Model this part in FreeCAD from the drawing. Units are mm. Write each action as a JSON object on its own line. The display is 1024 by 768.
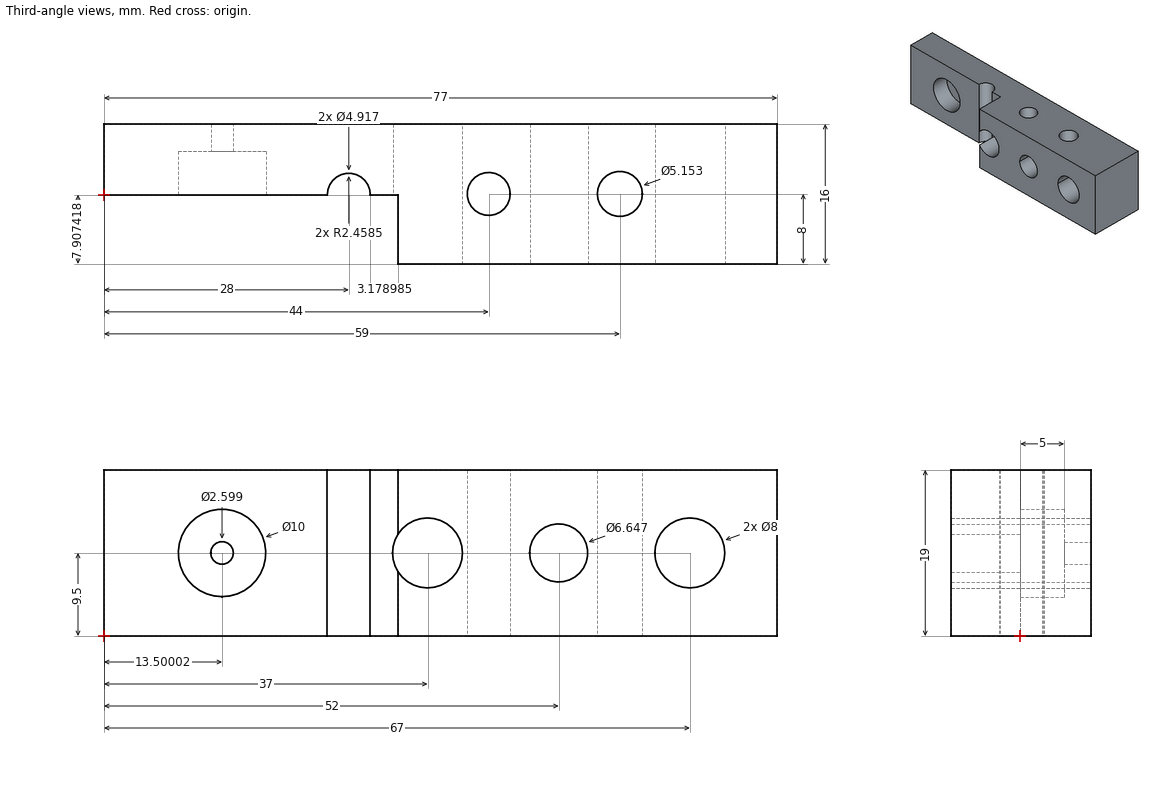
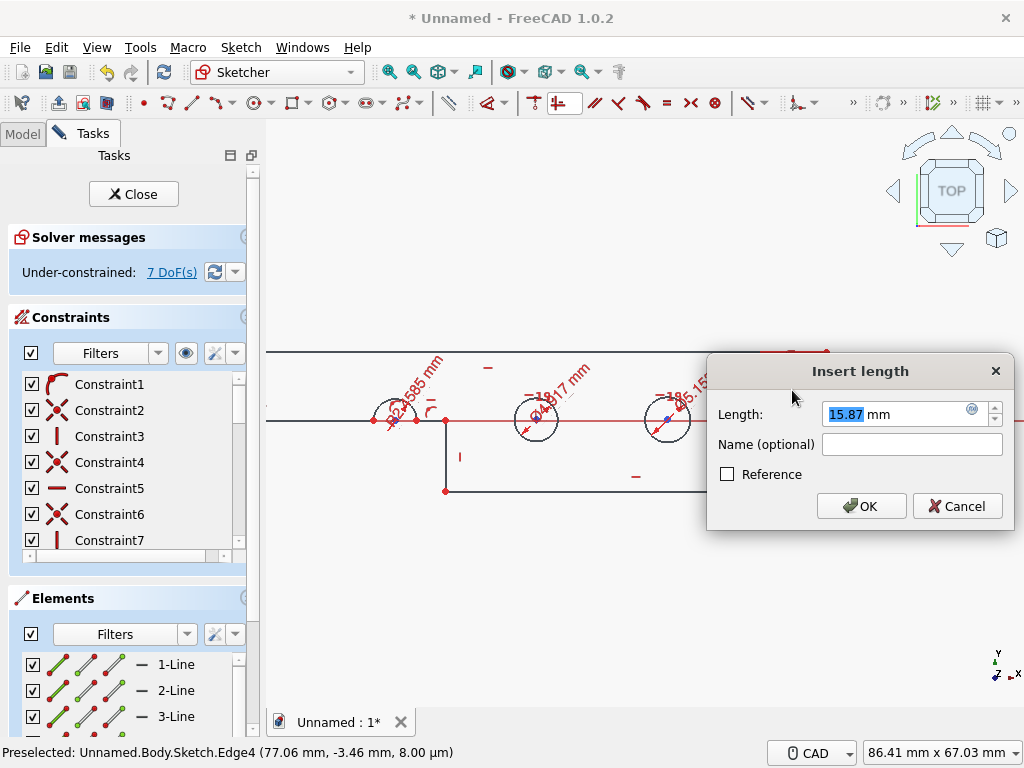
{"action": "type", "text": "16"}
{"action": "key", "text": "Return"}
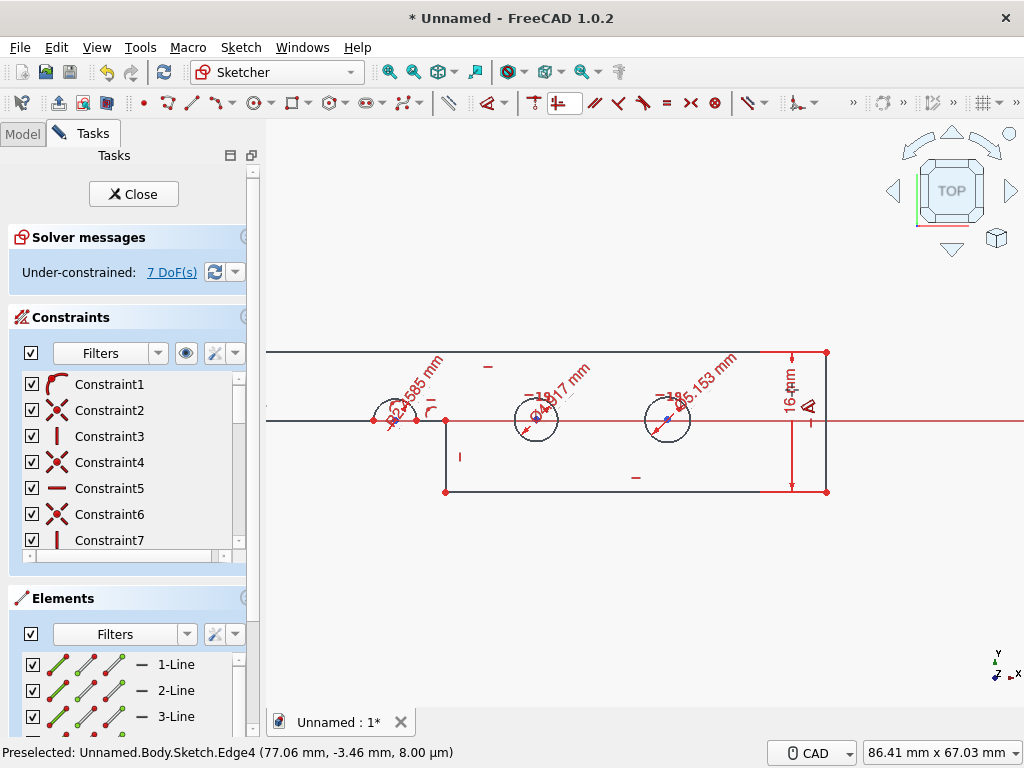
{"action": "left_click", "coordinate": [623, 352]}
{"action": "left_click", "coordinate": [560, 318]}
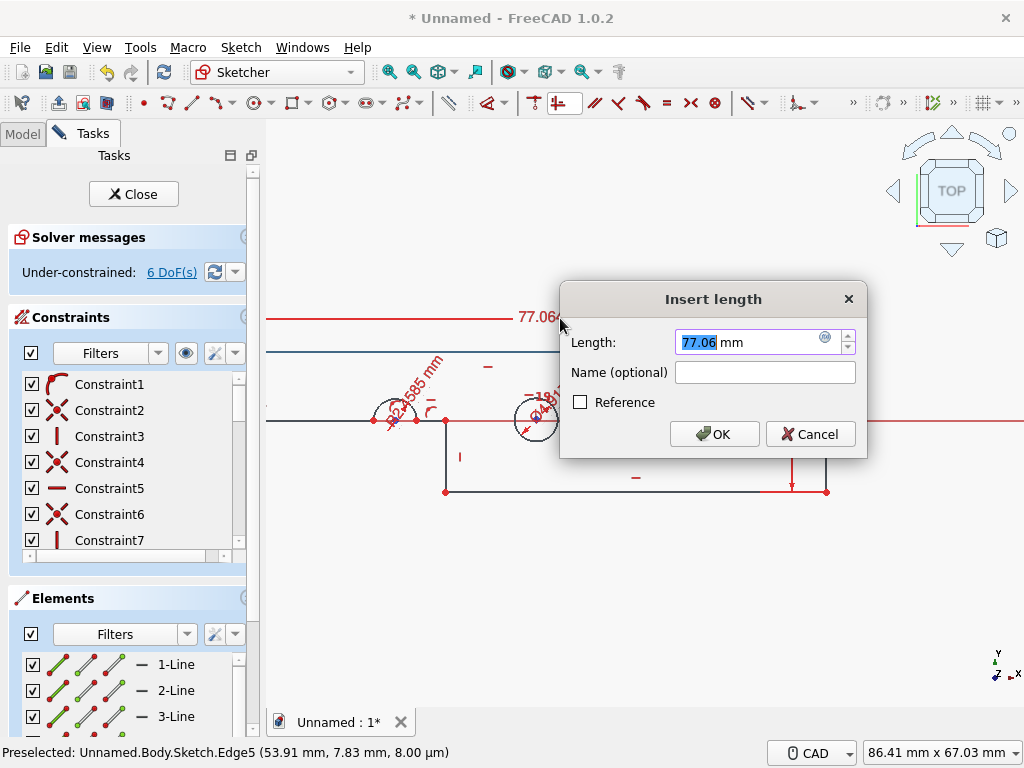
{"action": "type", "text": "77"}
{"action": "key", "text": "Return"}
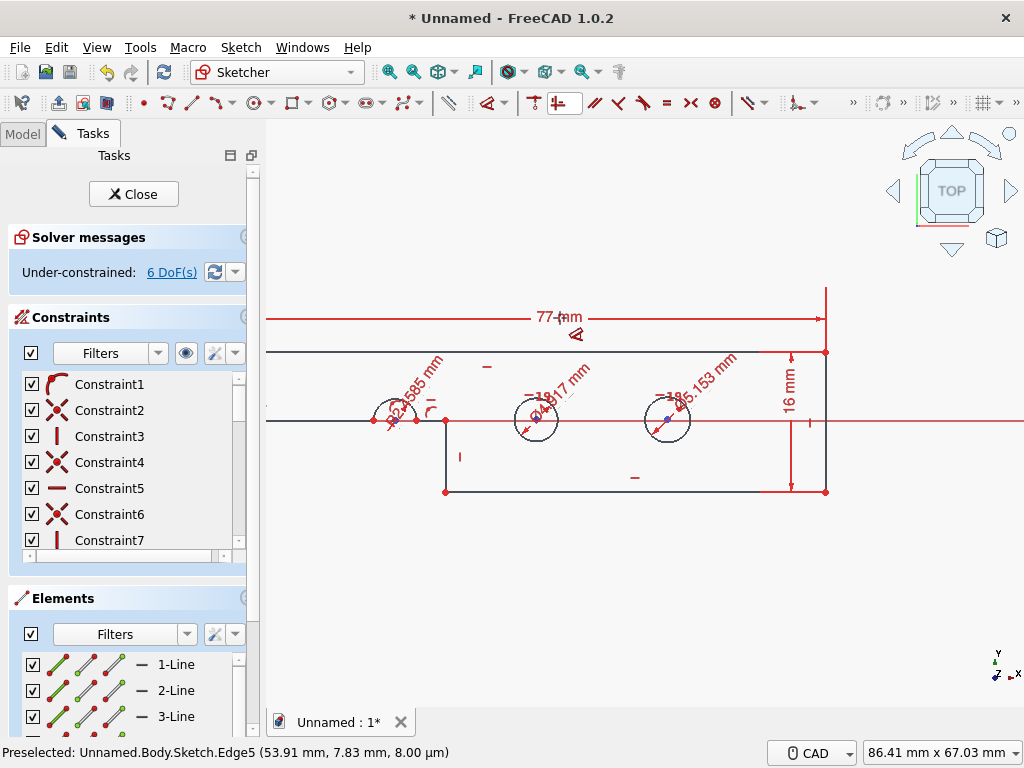
{"action": "left_click", "coordinate": [536, 420]}
{"action": "left_click", "coordinate": [415, 455]}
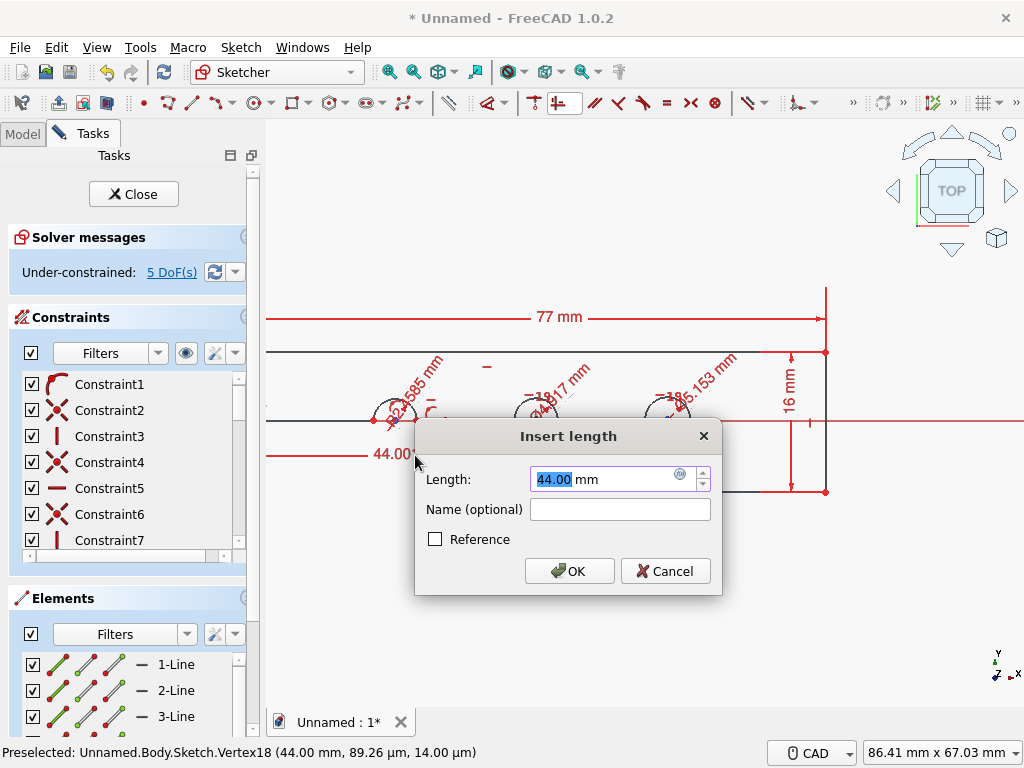
{"action": "type", "text": "44"}
{"action": "key", "text": "Return"}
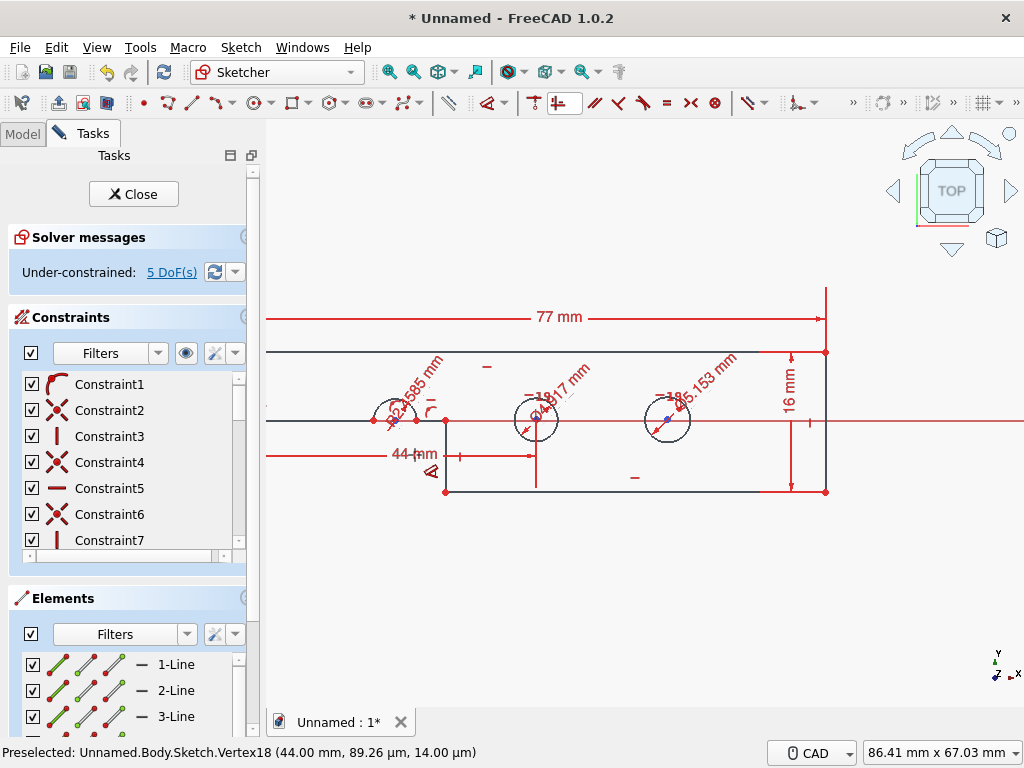
{"action": "left_click", "coordinate": [668, 420]}
{"action": "left_click", "coordinate": [567, 455]}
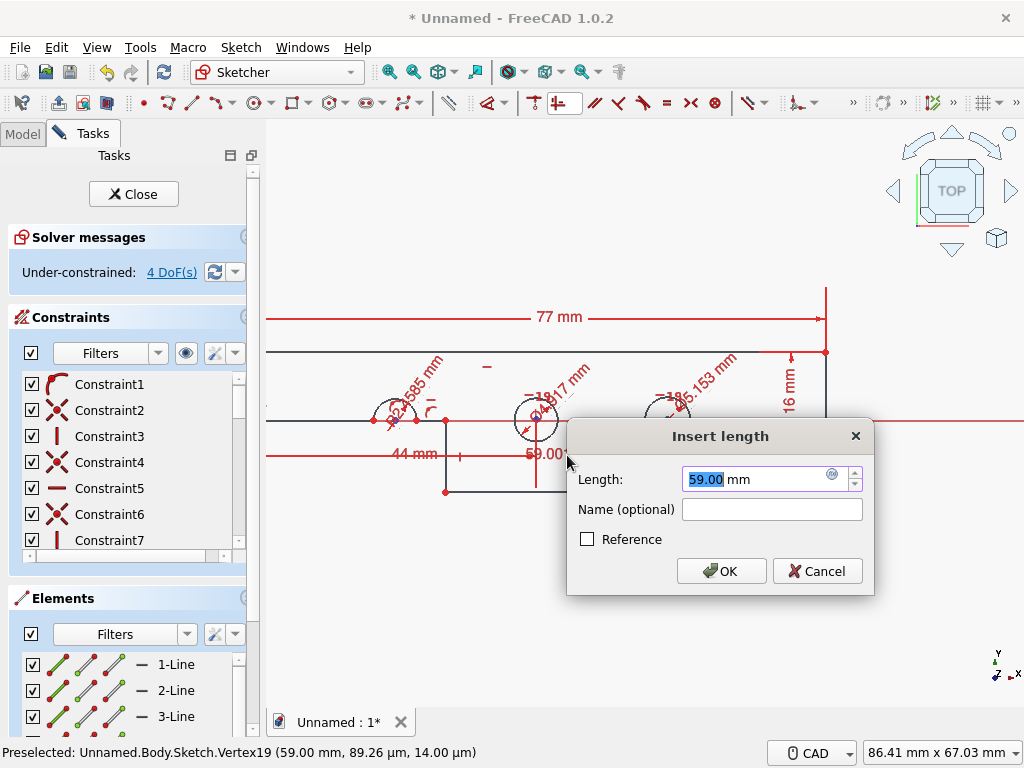
{"action": "type", "text": "59"}
{"action": "key", "text": "Return"}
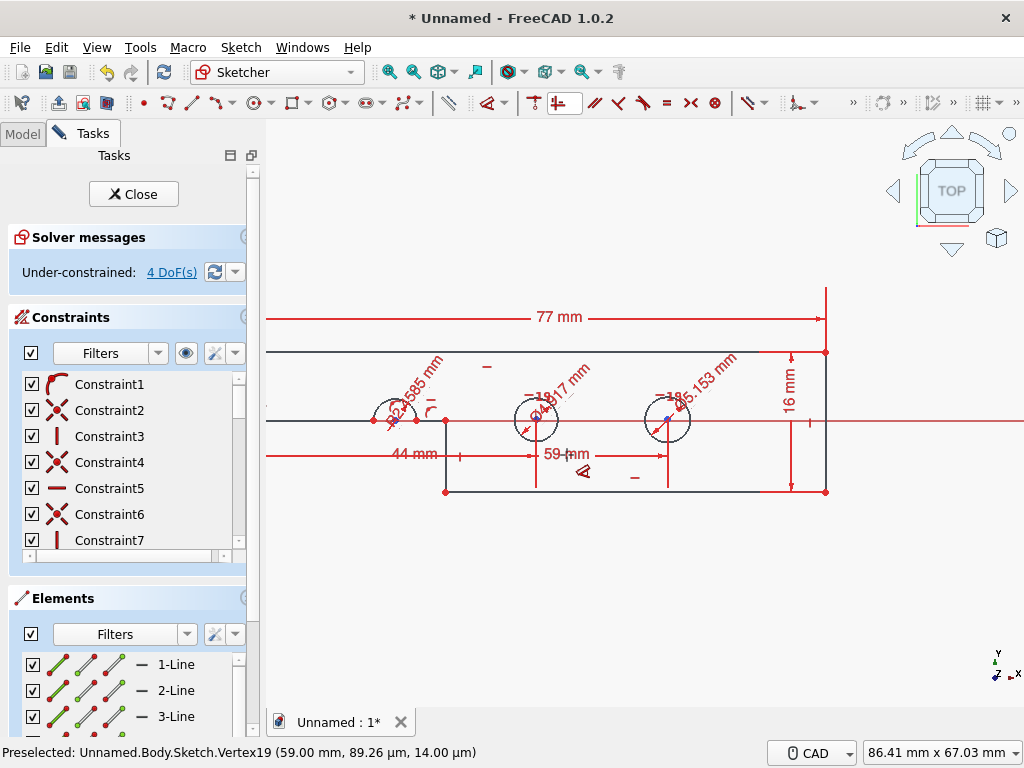
{"action": "left_click", "coordinate": [446, 492]}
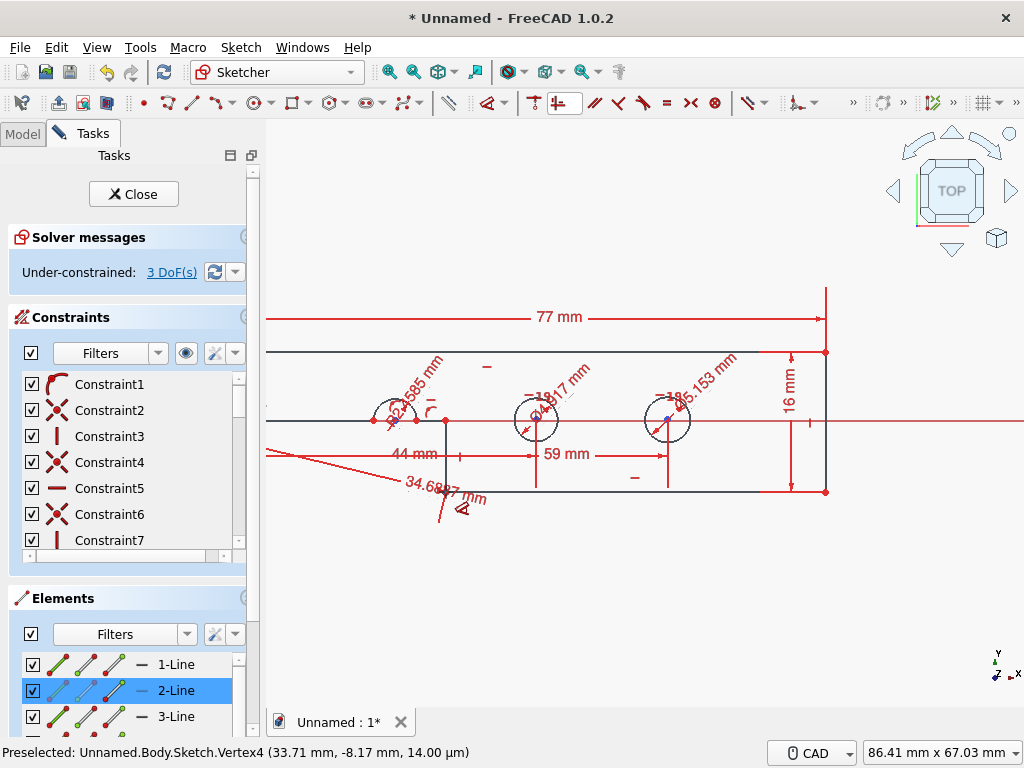
{"action": "left_click", "coordinate": [536, 420]}
{"action": "left_click", "coordinate": [412, 481]}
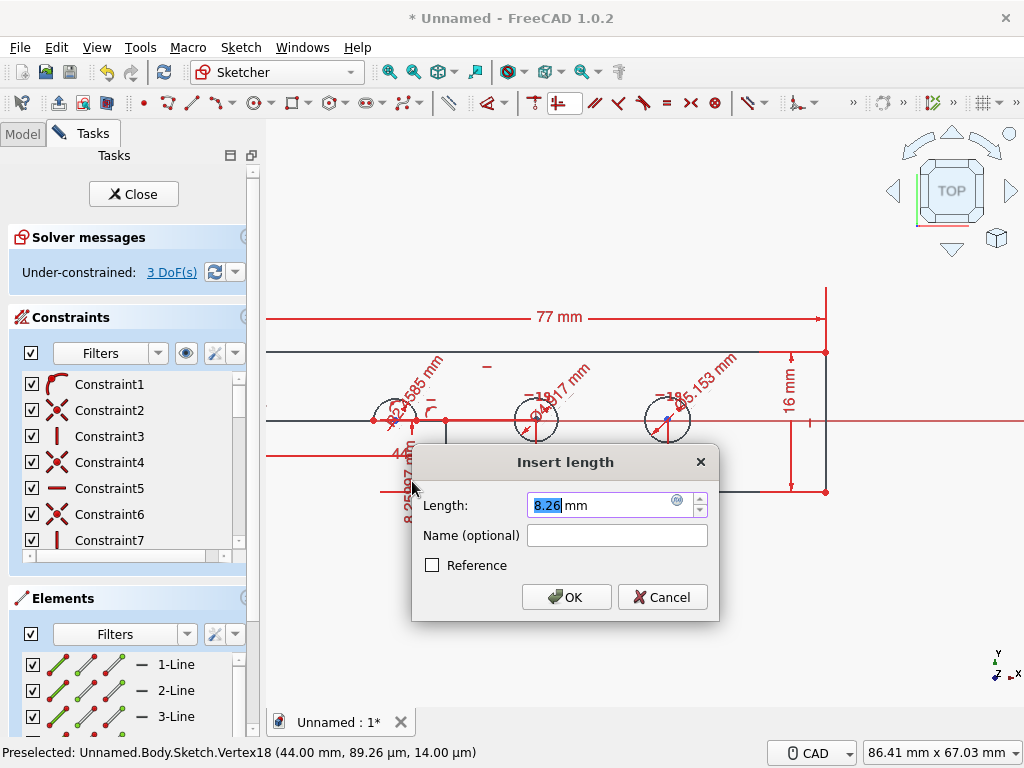
{"action": "type", "text": "8"}
{"action": "key", "text": "Return"}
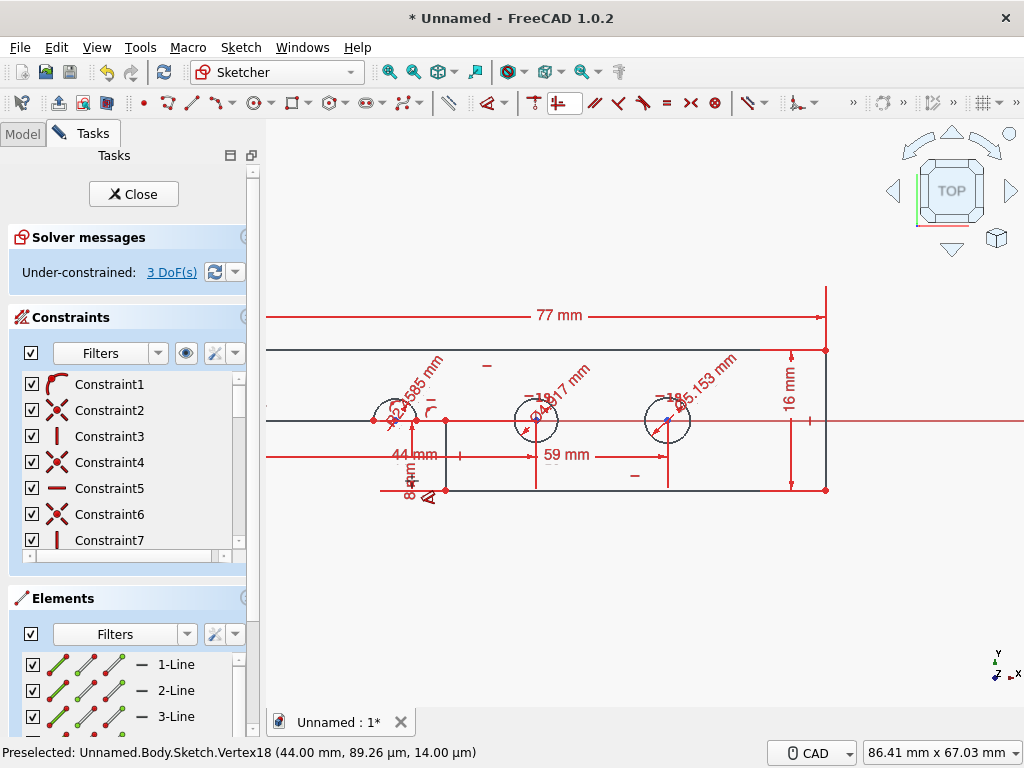
{"action": "left_click", "coordinate": [395, 421]}
{"action": "left_click", "coordinate": [345, 455]}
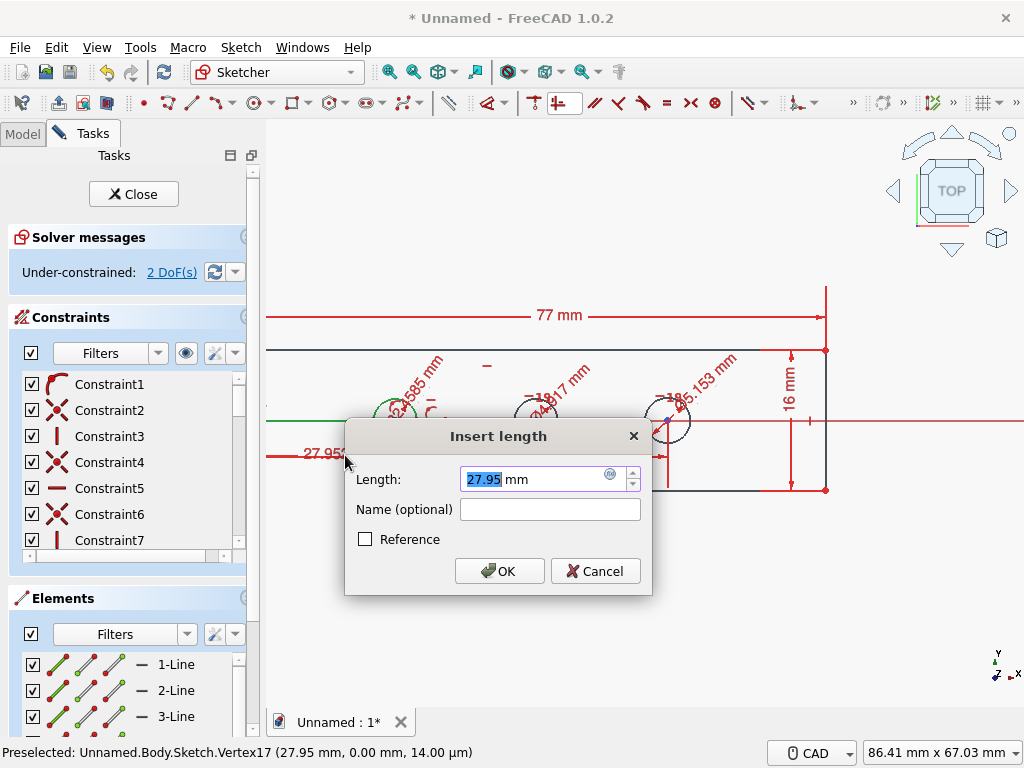
{"action": "type", "text": "28"}
{"action": "key", "text": "Return"}